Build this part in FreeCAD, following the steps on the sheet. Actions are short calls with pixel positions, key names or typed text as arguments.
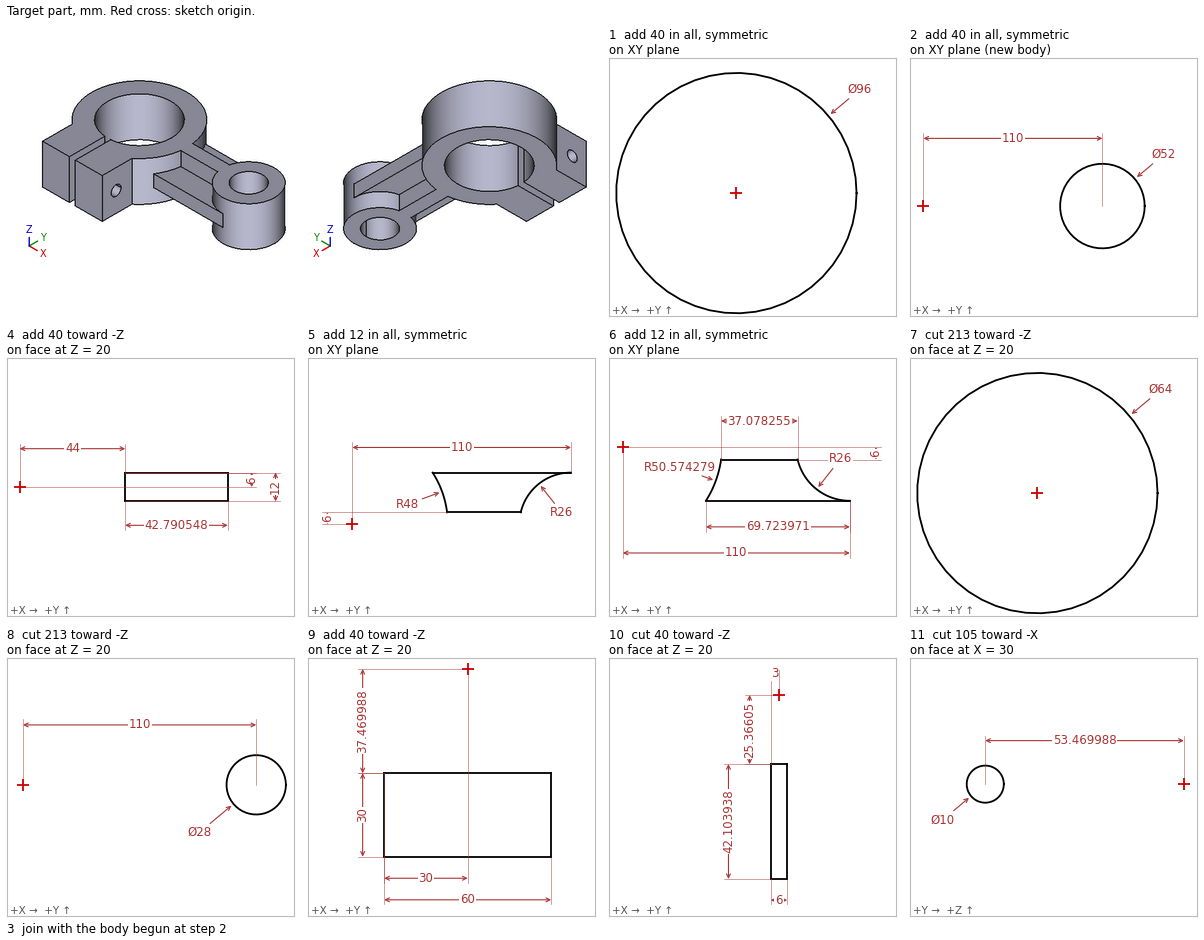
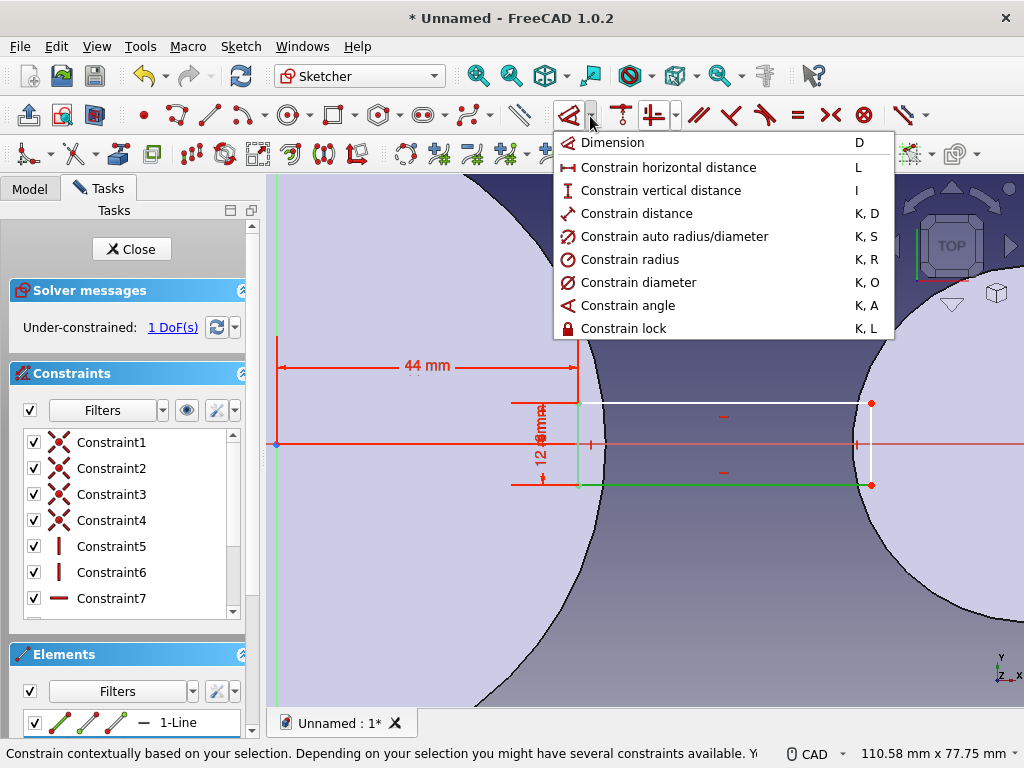
click(724, 168)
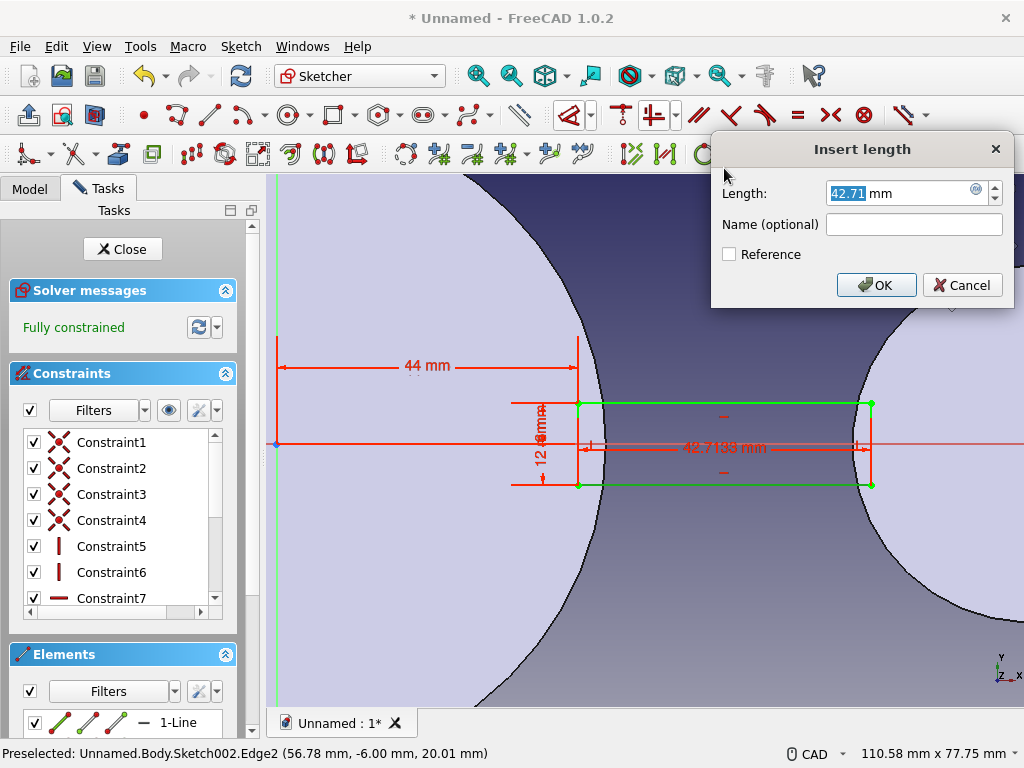
text(42.790548)
key(Return)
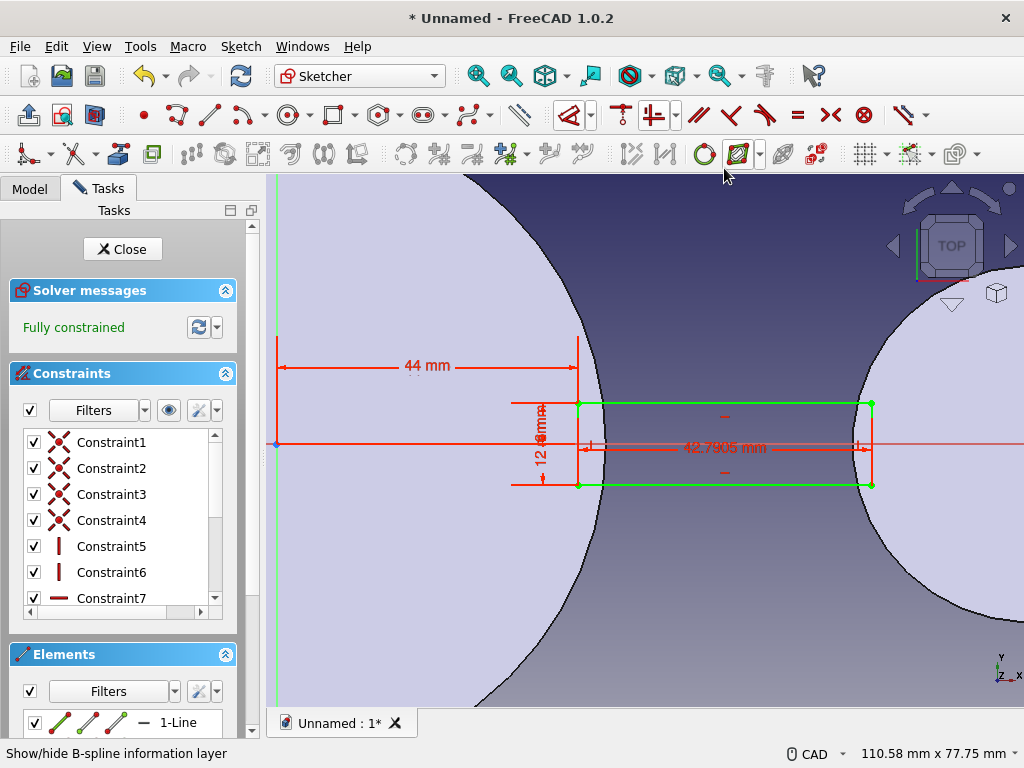
click(123, 249)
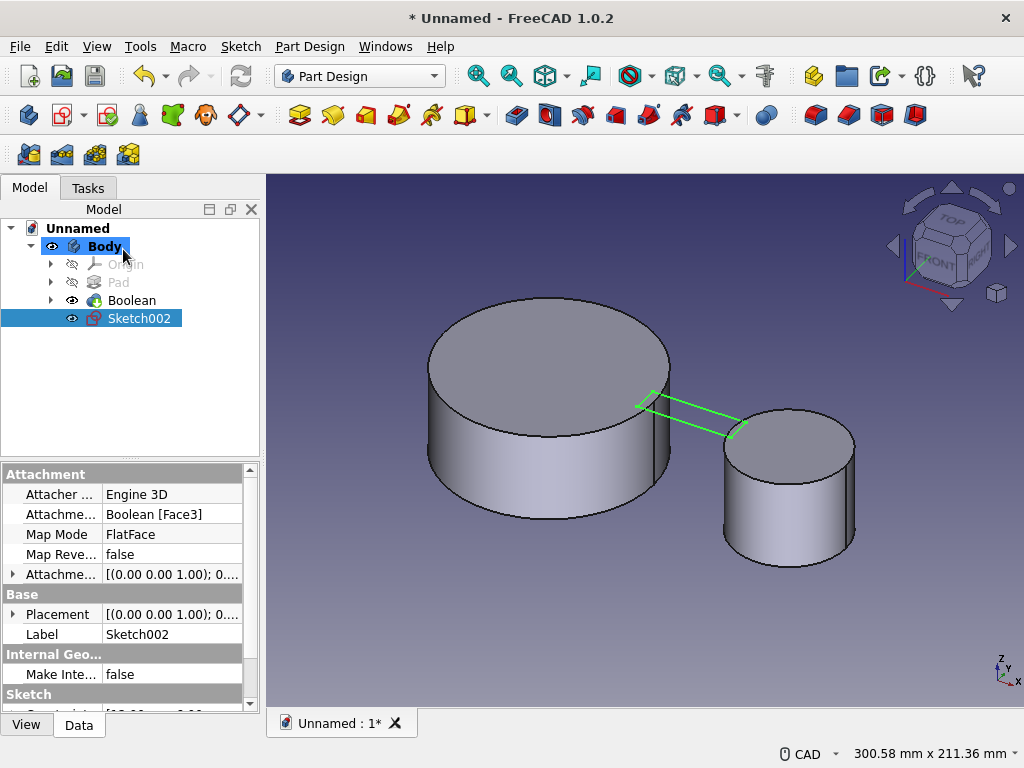
click(300, 116)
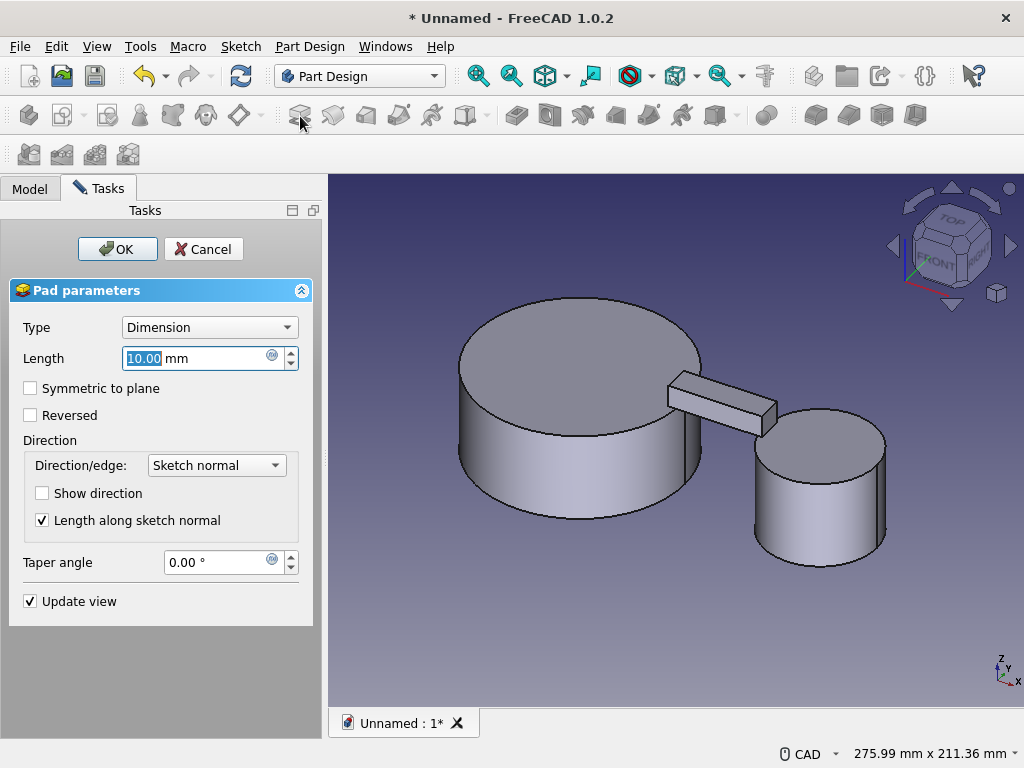
text(40)
key(Tab)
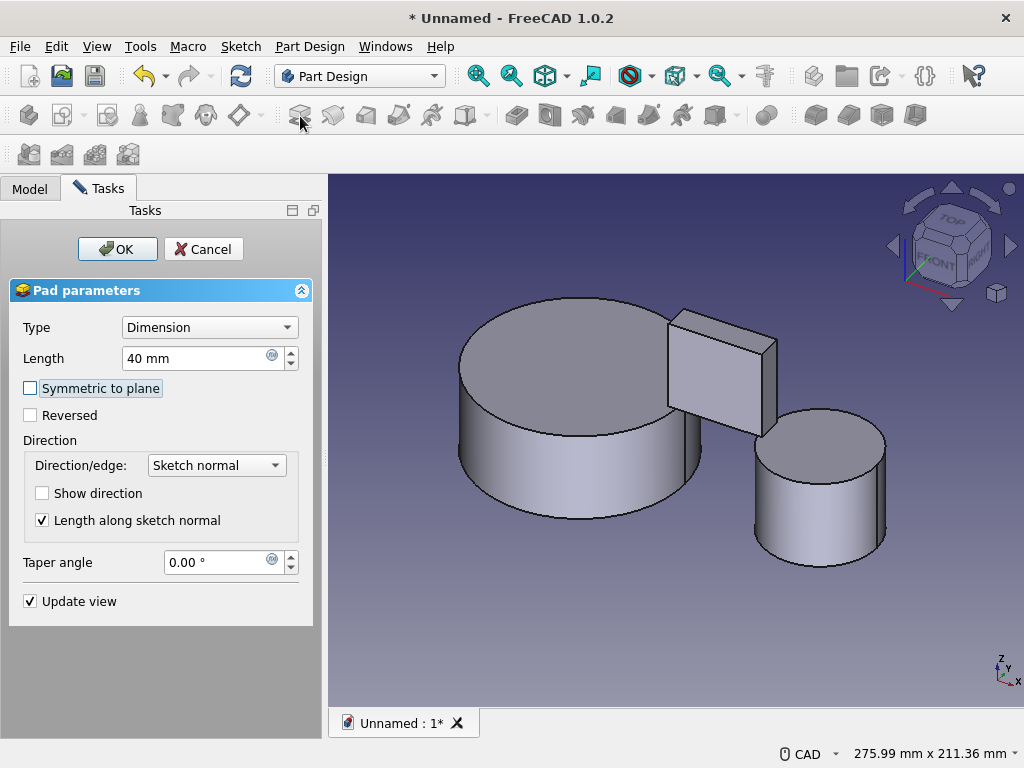
click(31, 415)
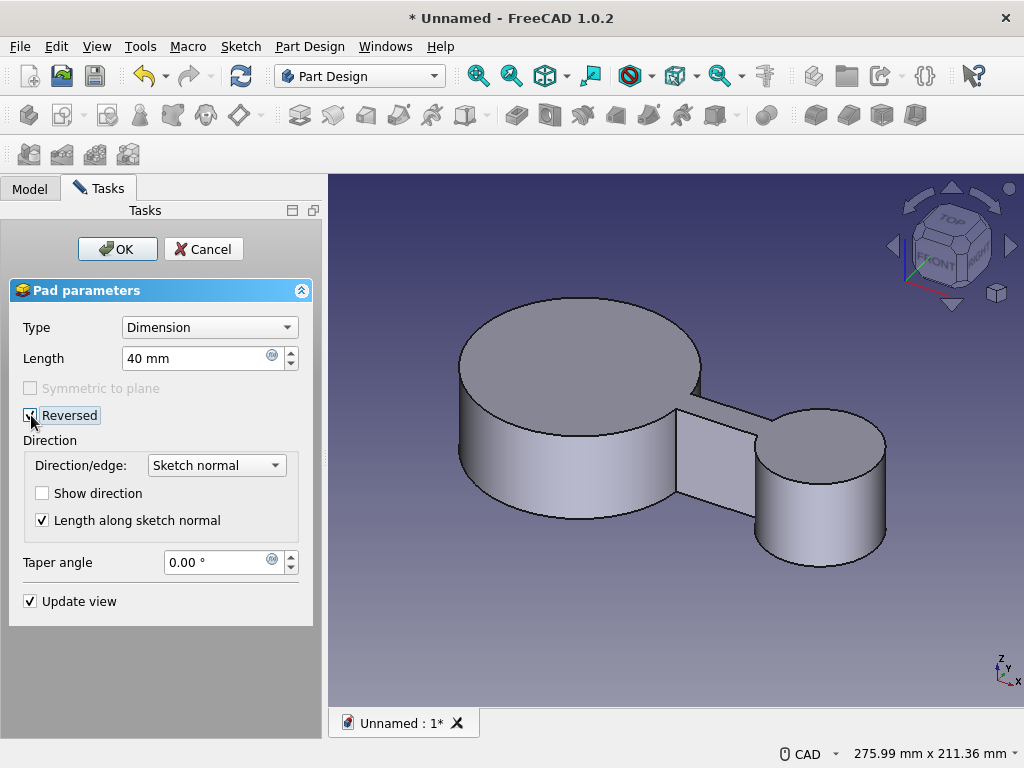
click(118, 249)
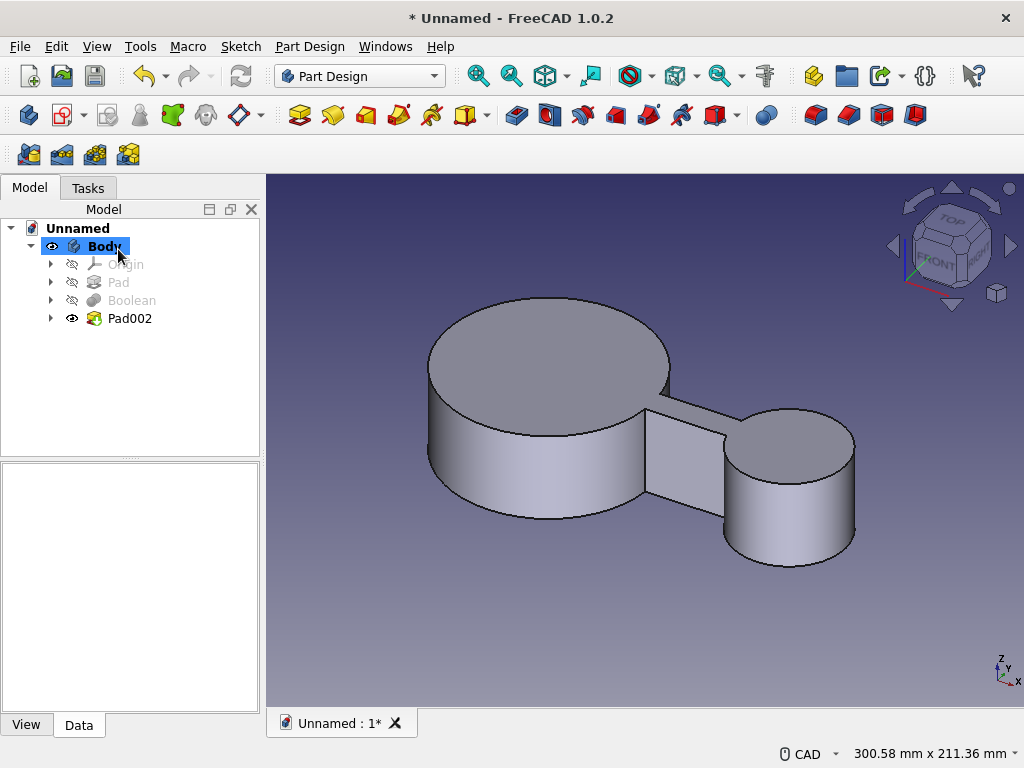
click(62, 116)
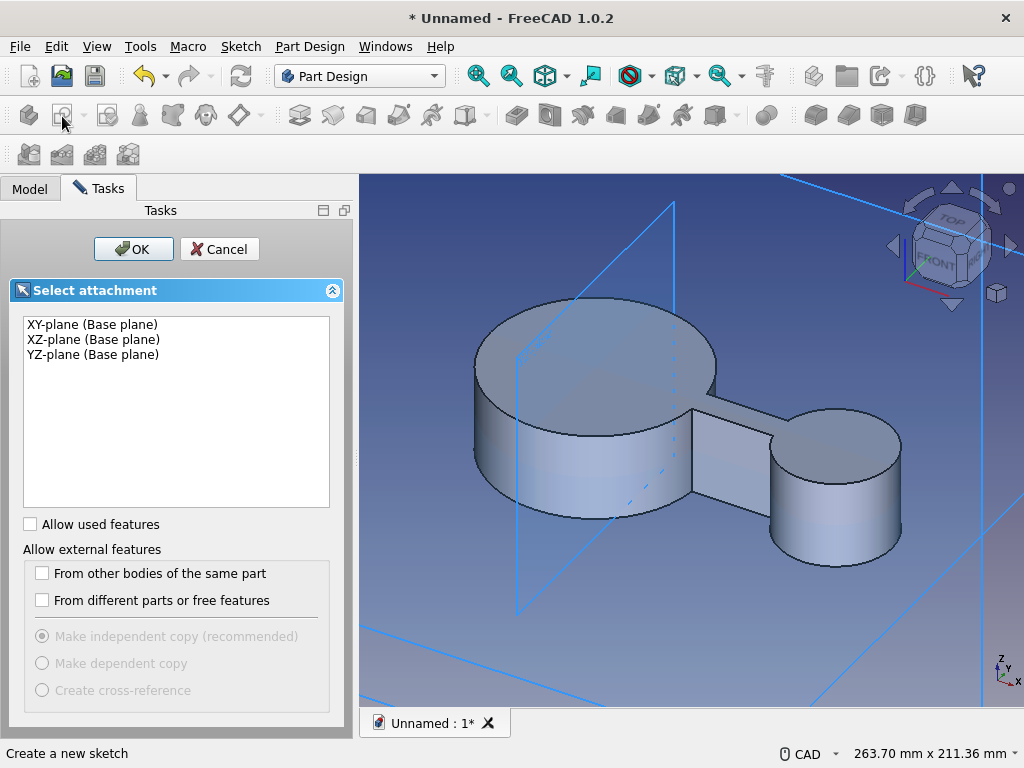
click(84, 324)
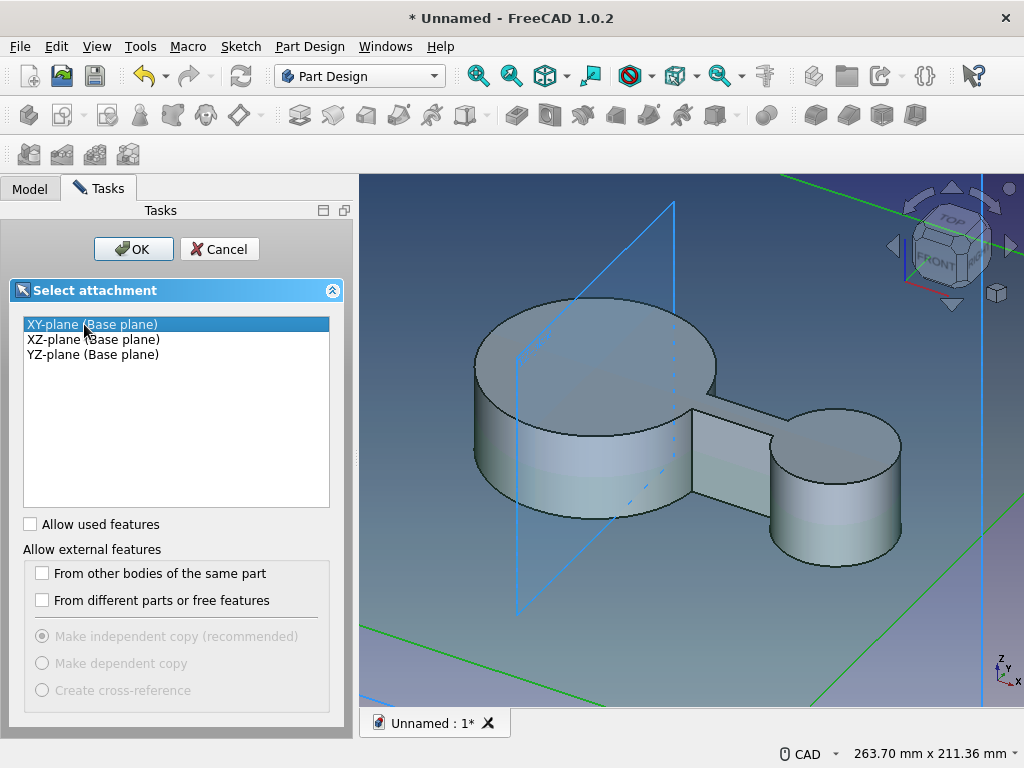
click(134, 249)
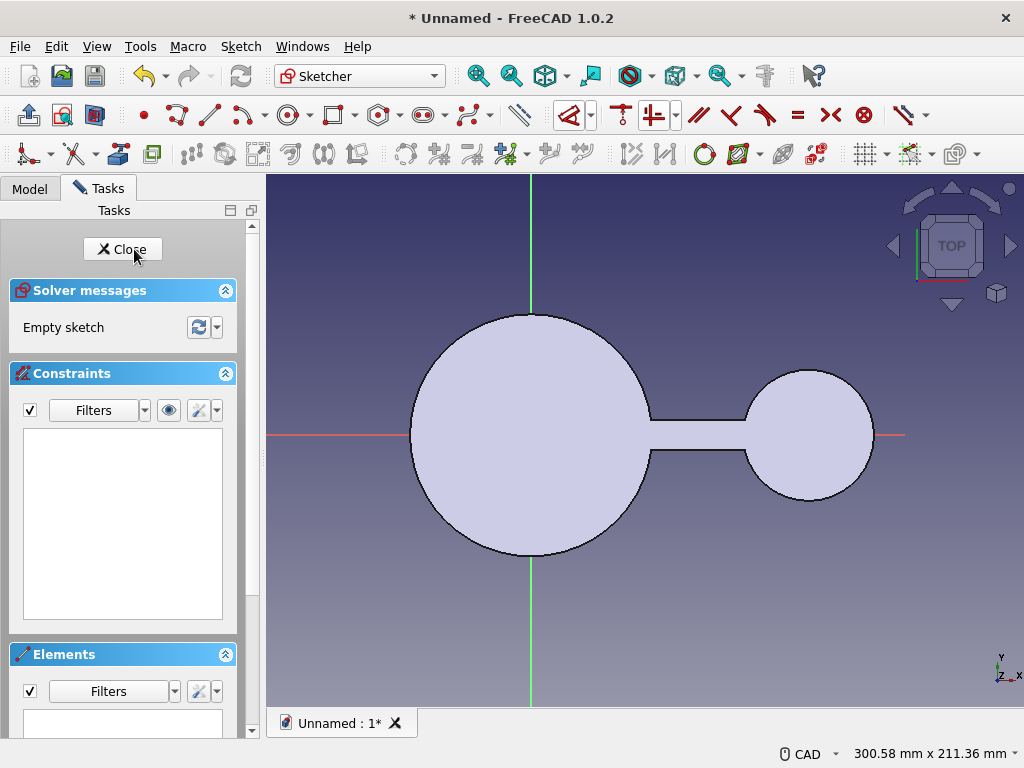
click(95, 116)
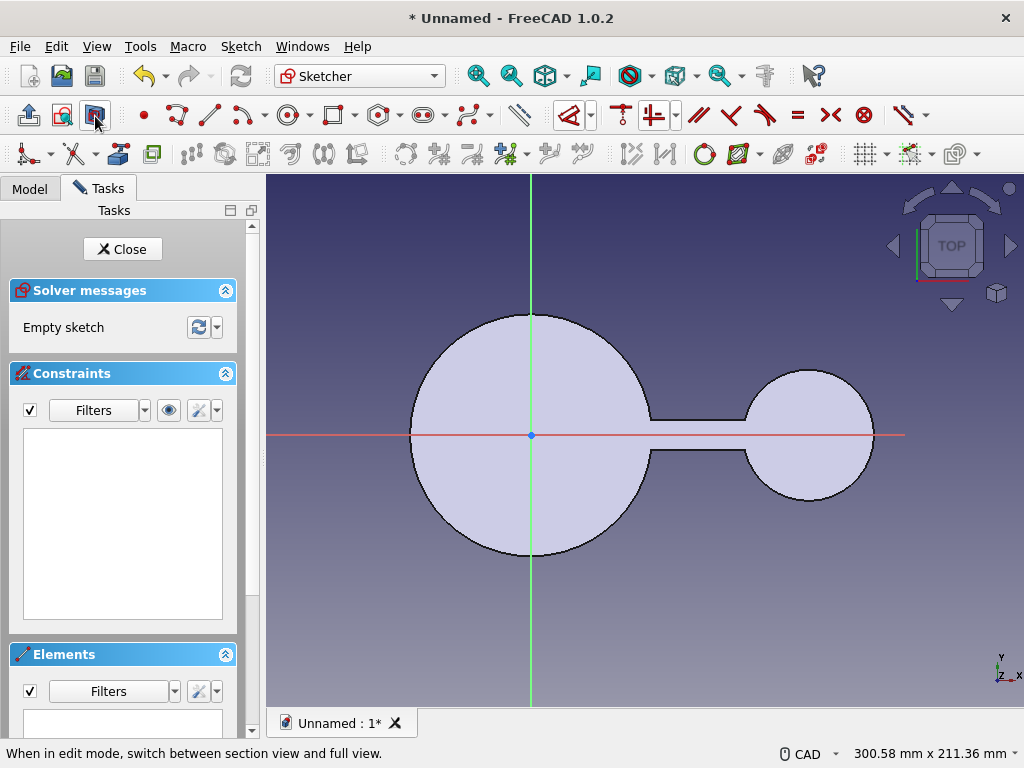
scroll(859, 325, up, 2)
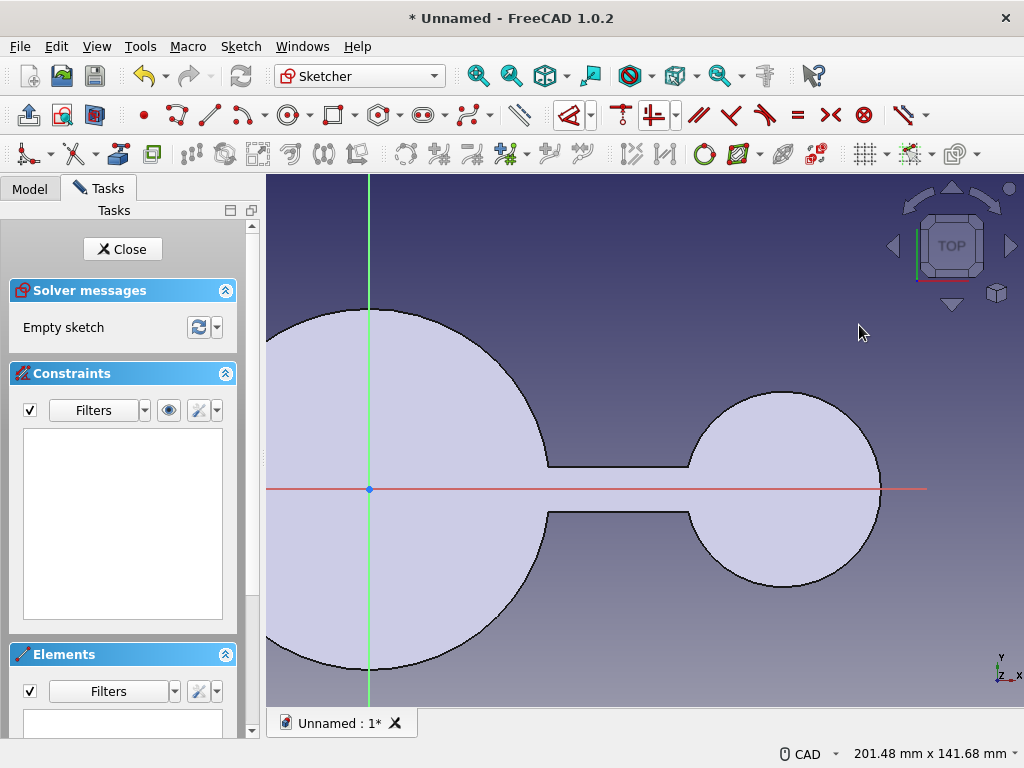
click(210, 116)